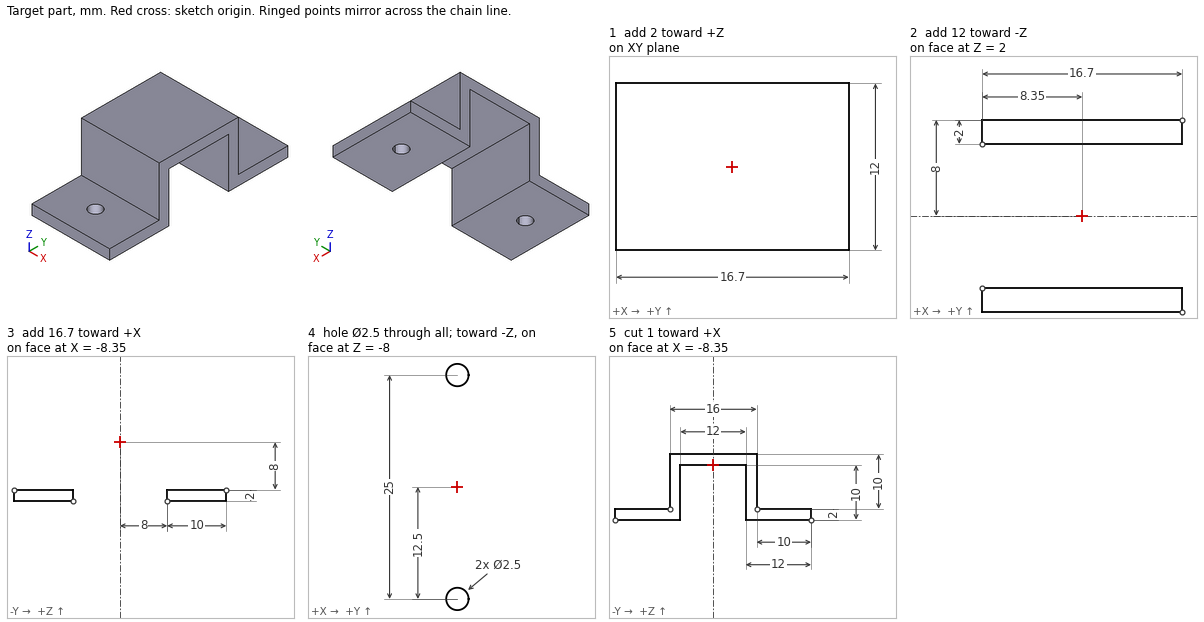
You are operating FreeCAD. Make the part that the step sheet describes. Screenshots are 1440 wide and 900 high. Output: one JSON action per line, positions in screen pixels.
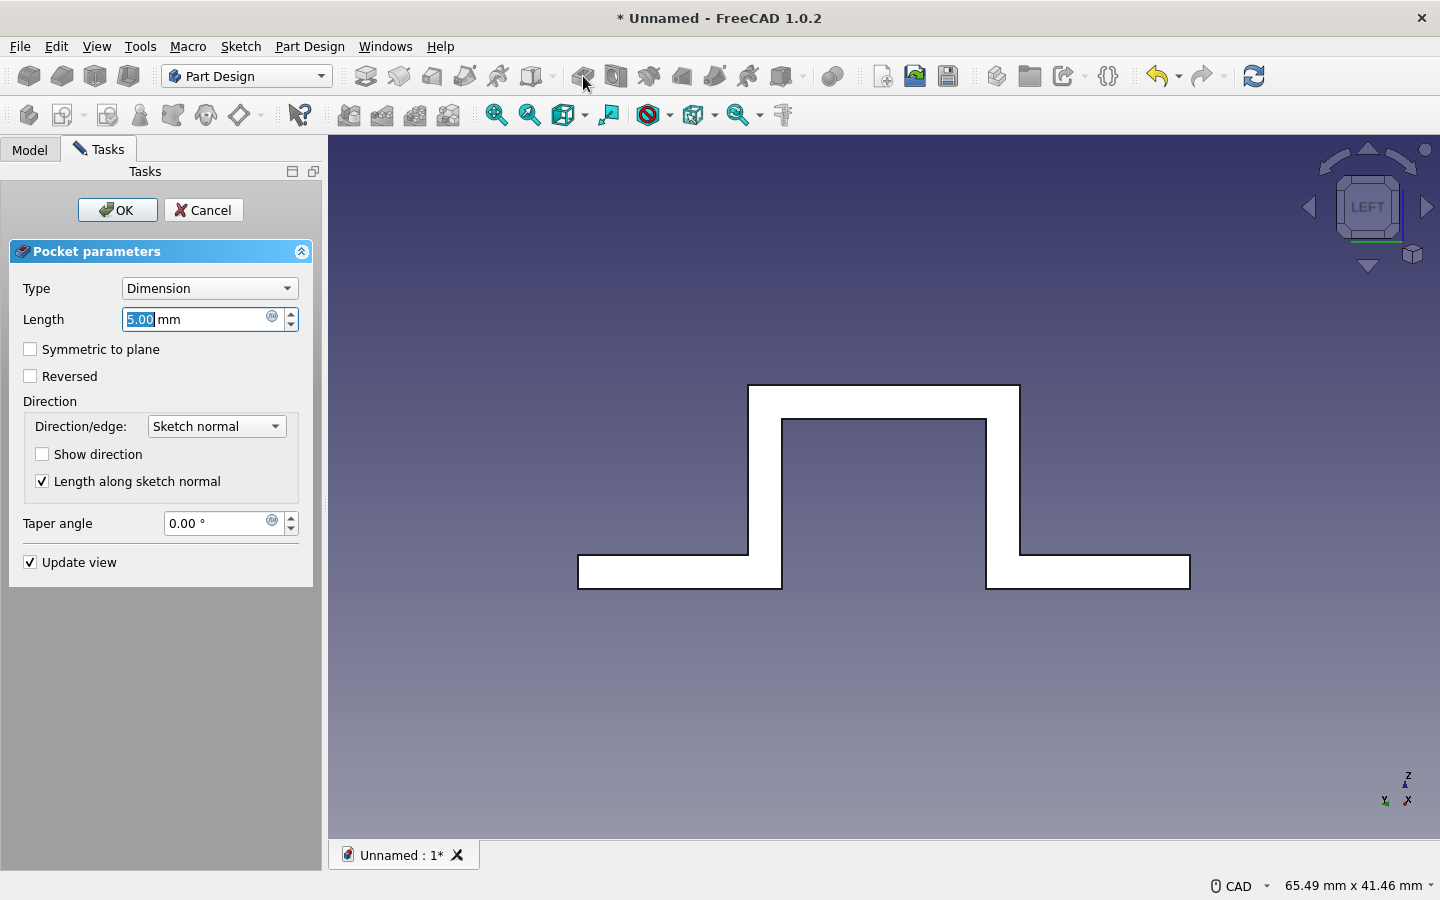
{"action": "type", "text": "1"}
{"action": "key", "text": "Tab"}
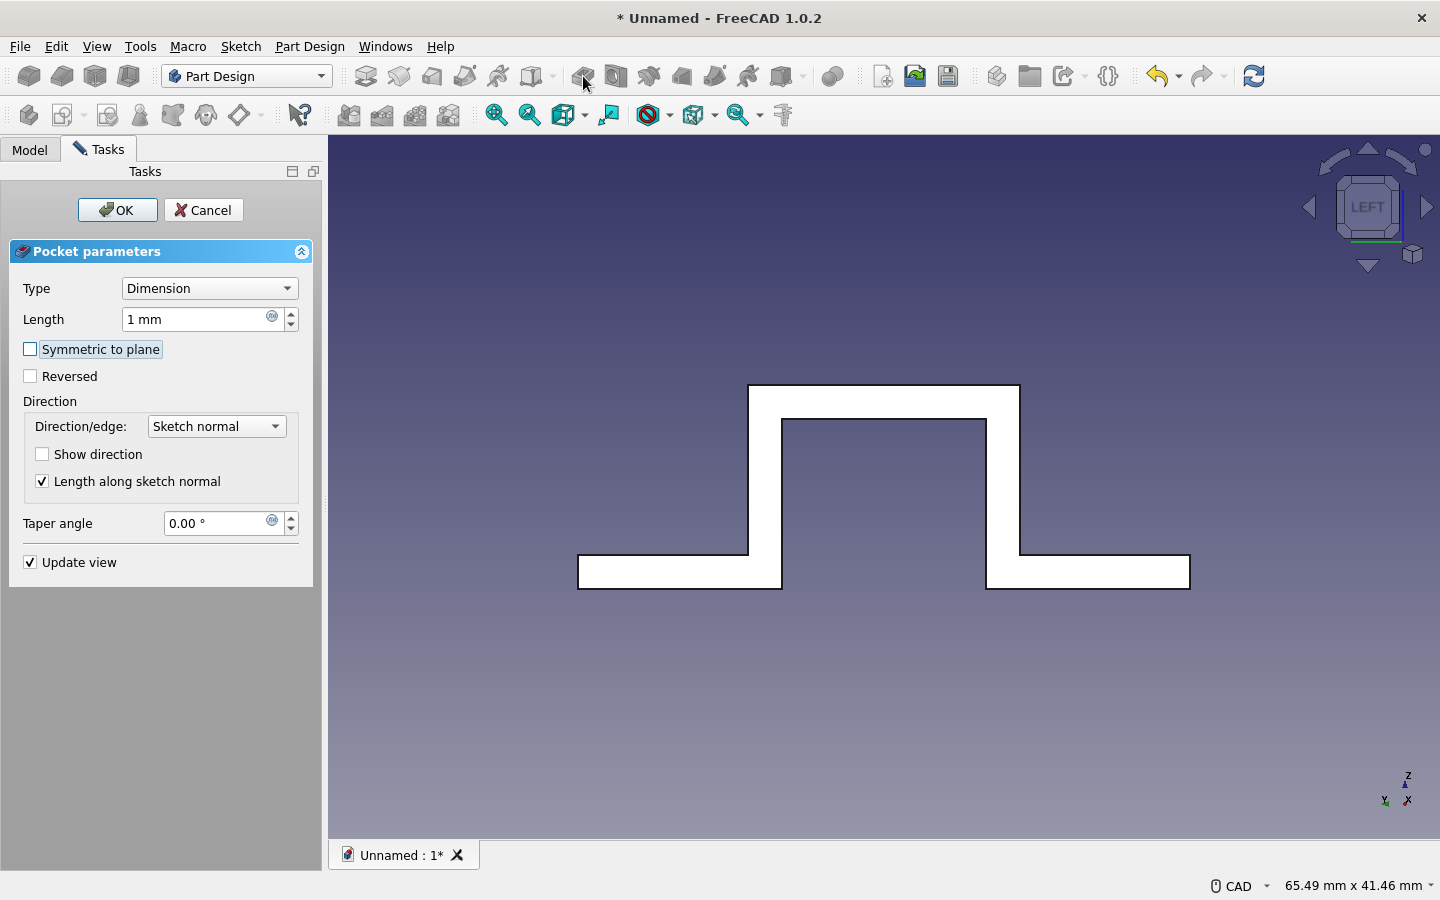
{"action": "left_click", "coordinate": [118, 210]}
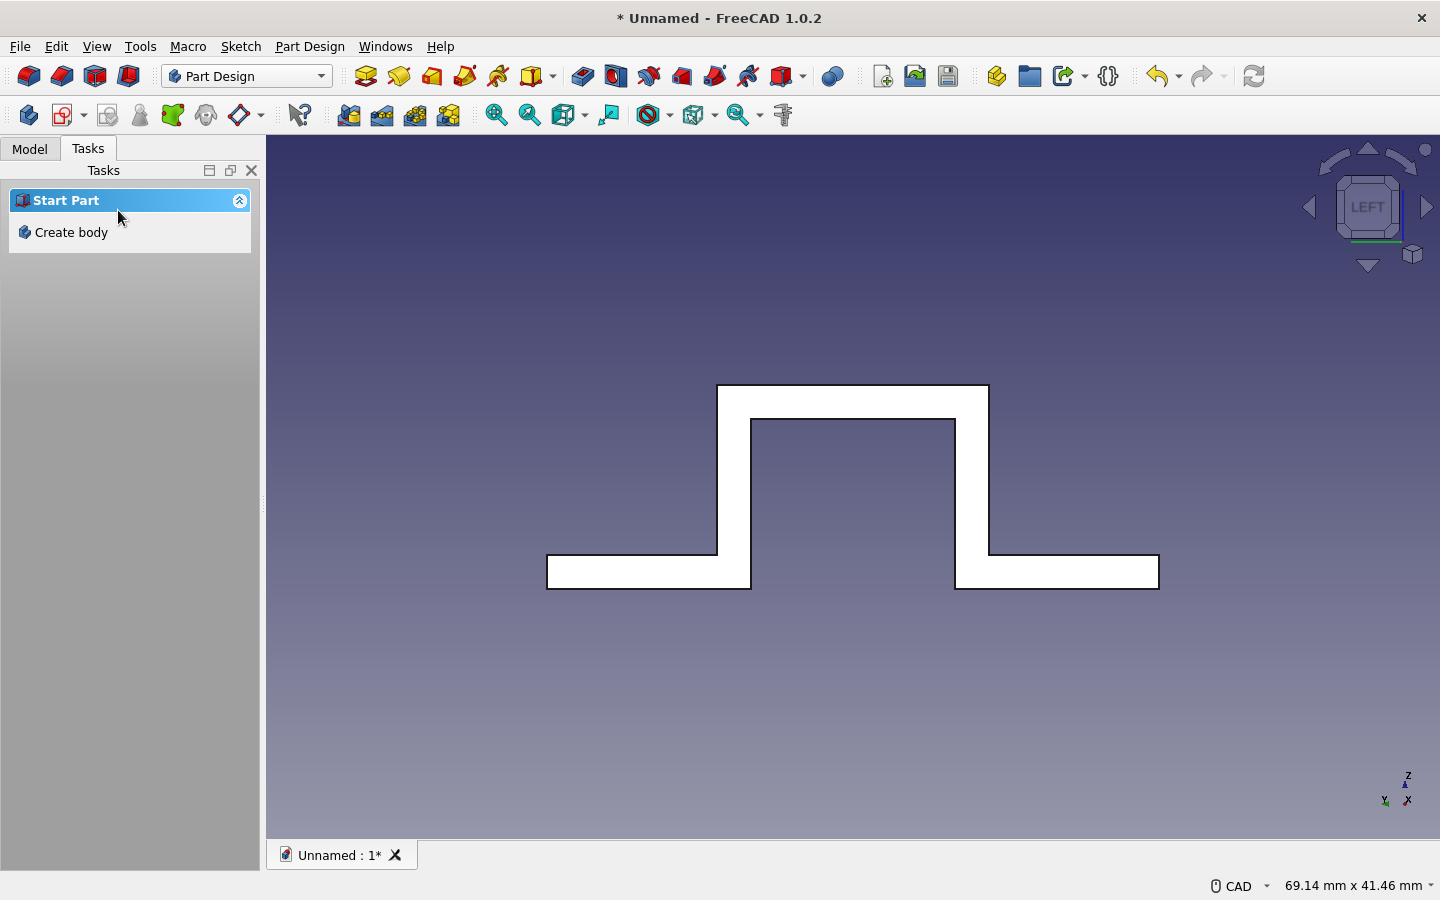
{"action": "key", "text": "0"}